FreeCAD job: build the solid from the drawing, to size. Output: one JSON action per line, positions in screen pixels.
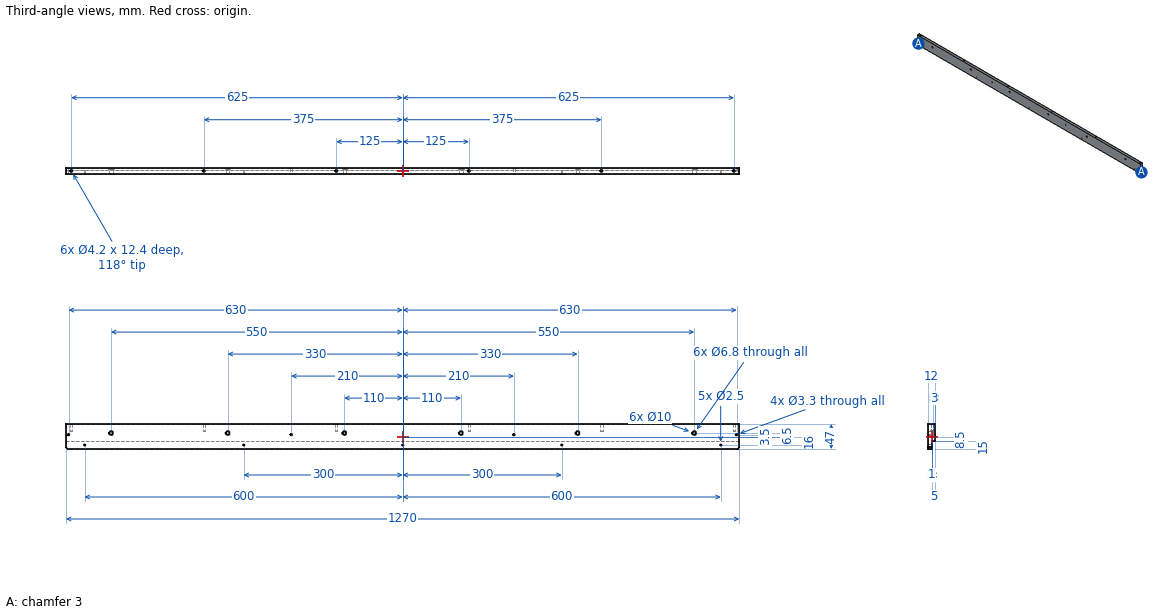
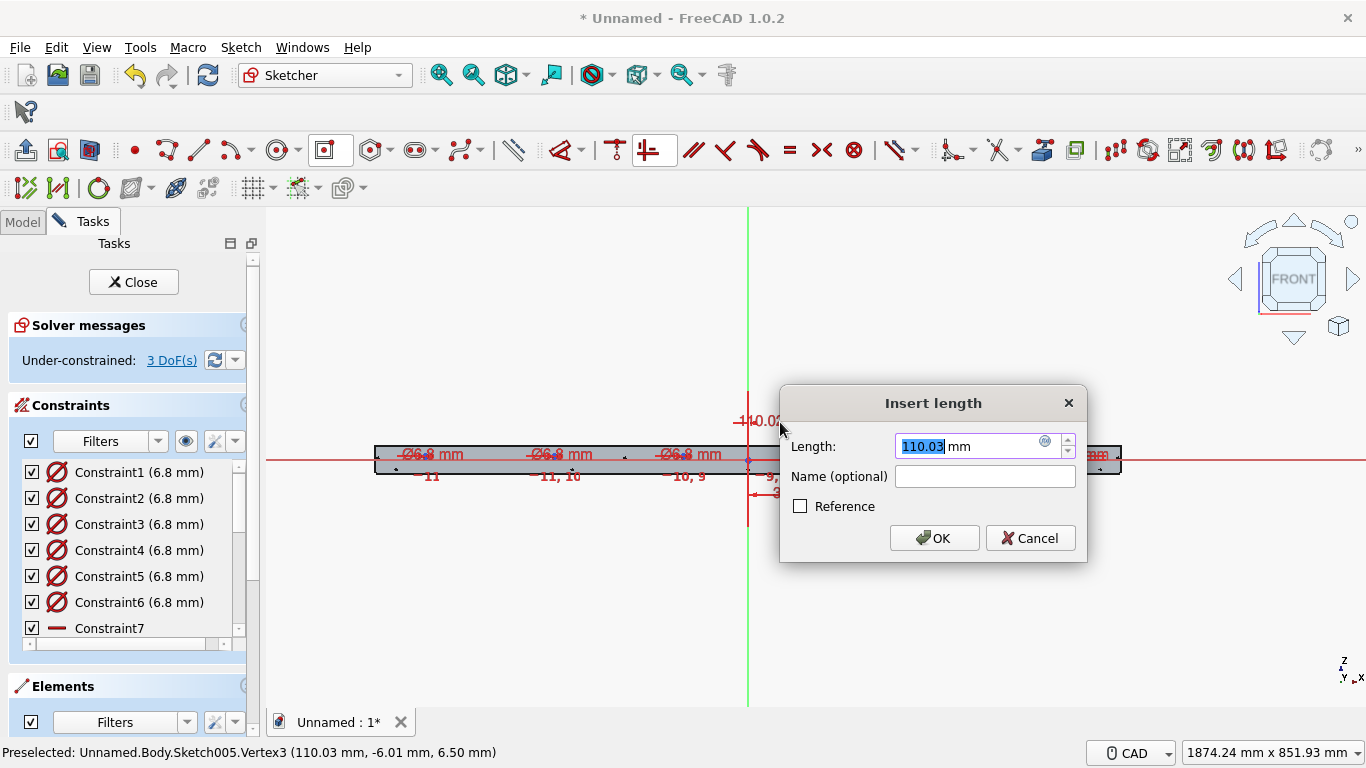
{"action": "type", "text": "110"}
{"action": "key", "text": "Return"}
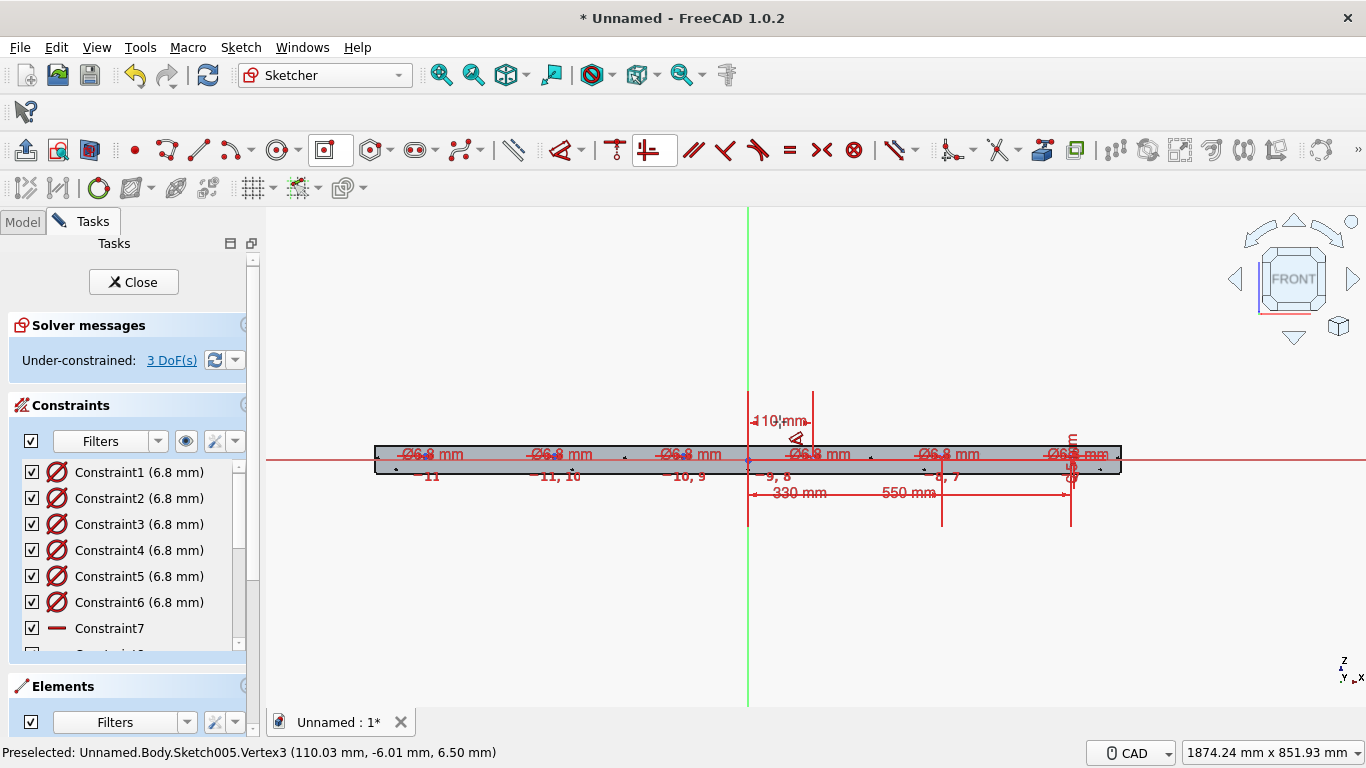
{"action": "left_click", "coordinate": [684, 456]}
{"action": "left_click", "coordinate": [716, 494]}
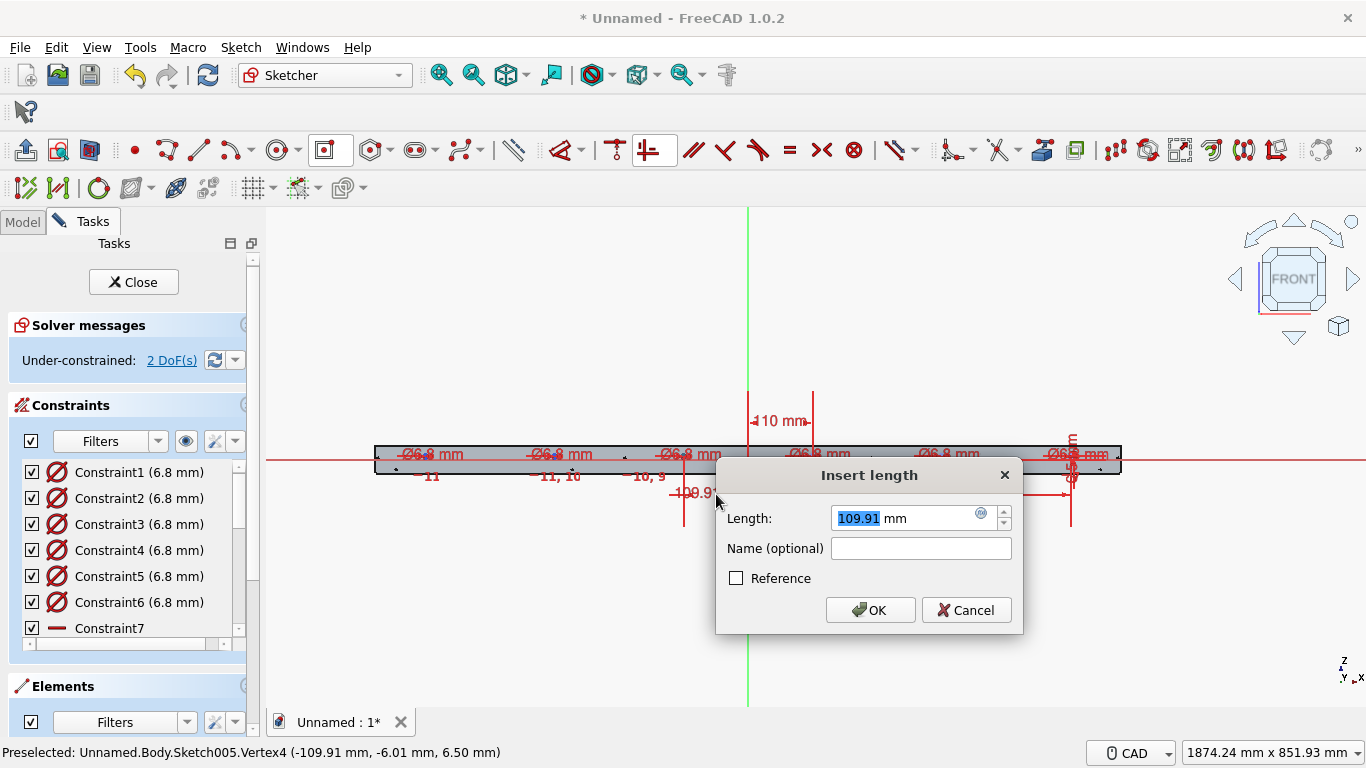
{"action": "type", "text": "110"}
{"action": "key", "text": "Return"}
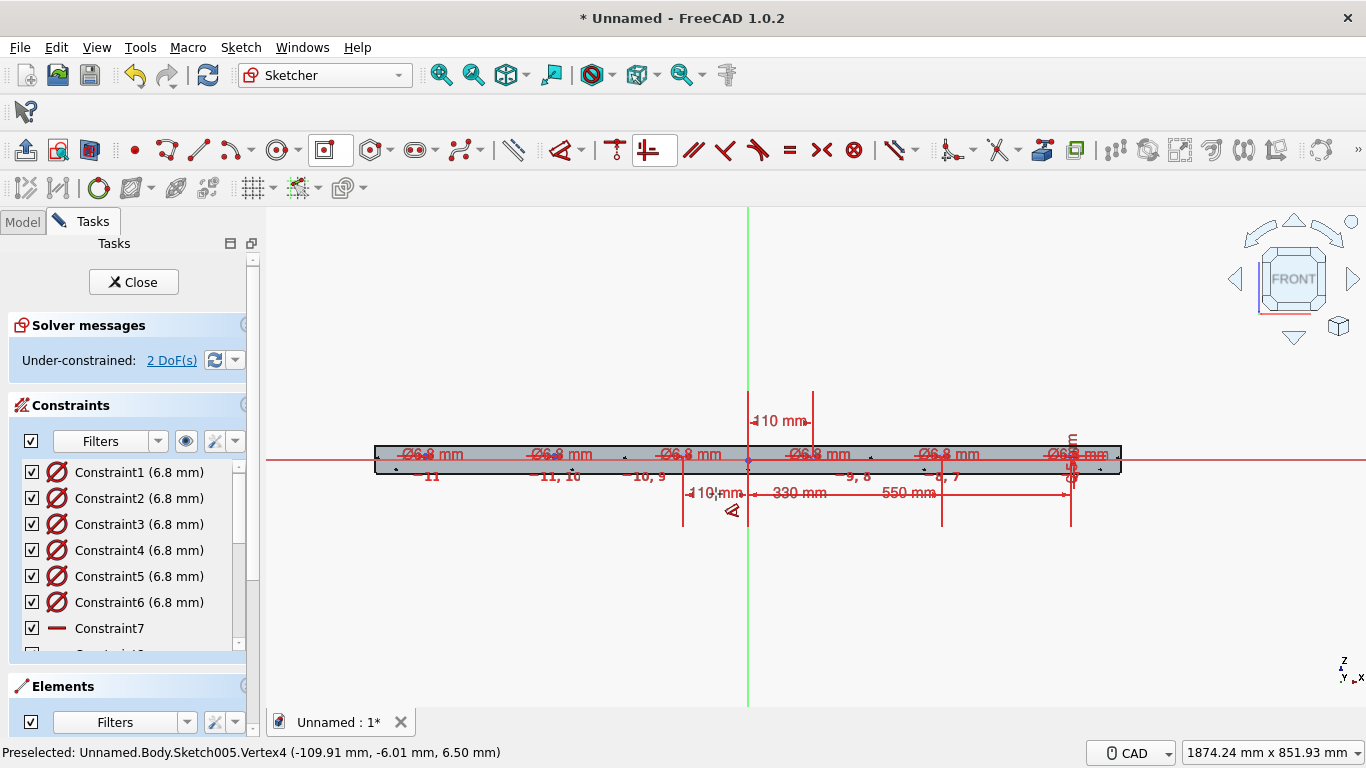
{"action": "left_click", "coordinate": [554, 456]}
{"action": "left_click", "coordinate": [607, 494]}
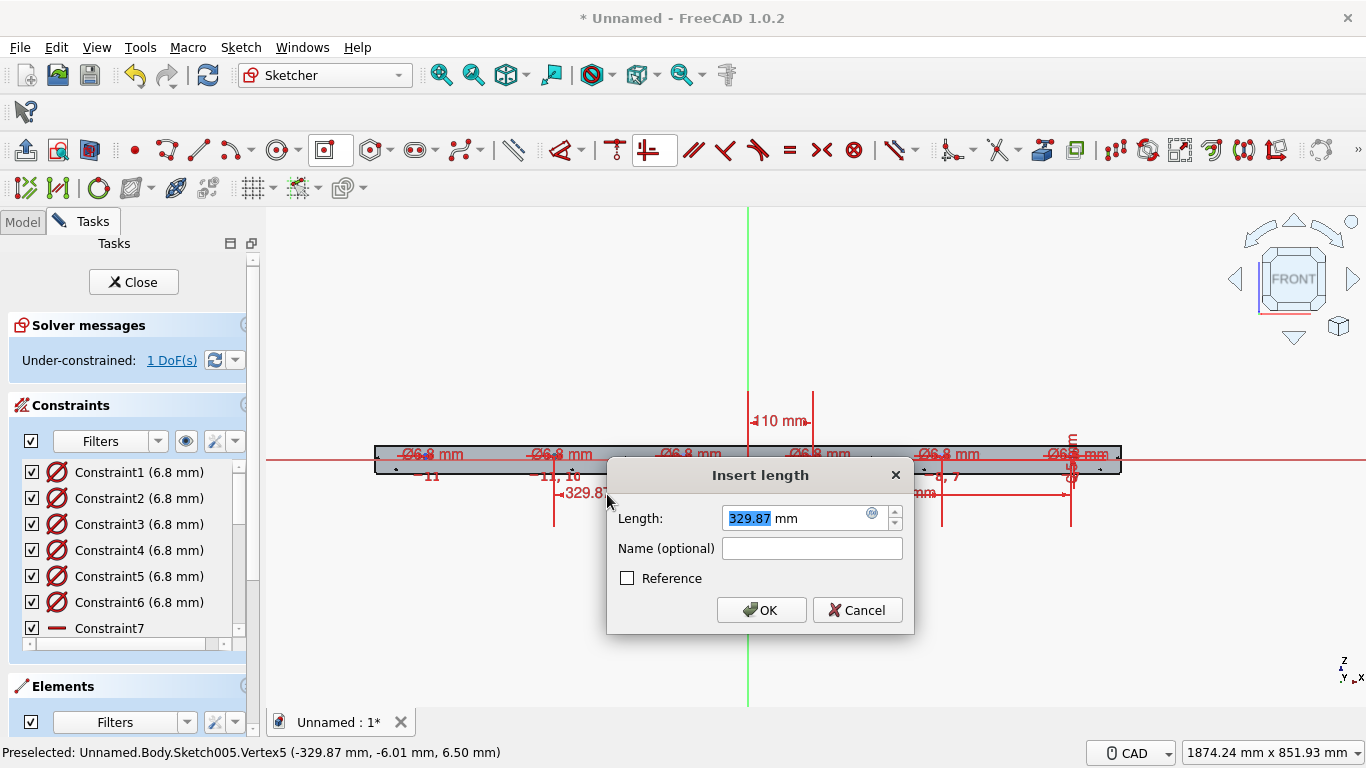
{"action": "type", "text": "330"}
{"action": "key", "text": "Return"}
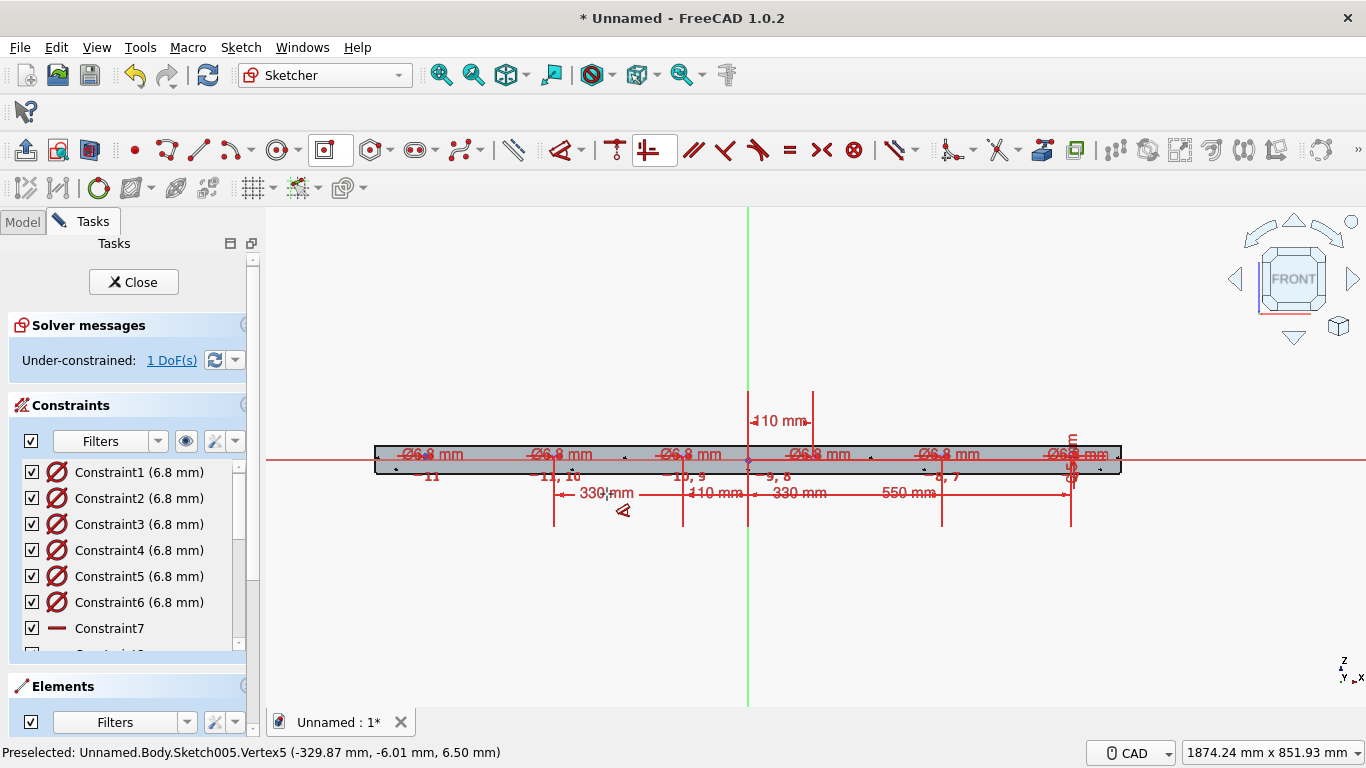
{"action": "left_click", "coordinate": [425, 456]}
{"action": "left_click", "coordinate": [512, 494]}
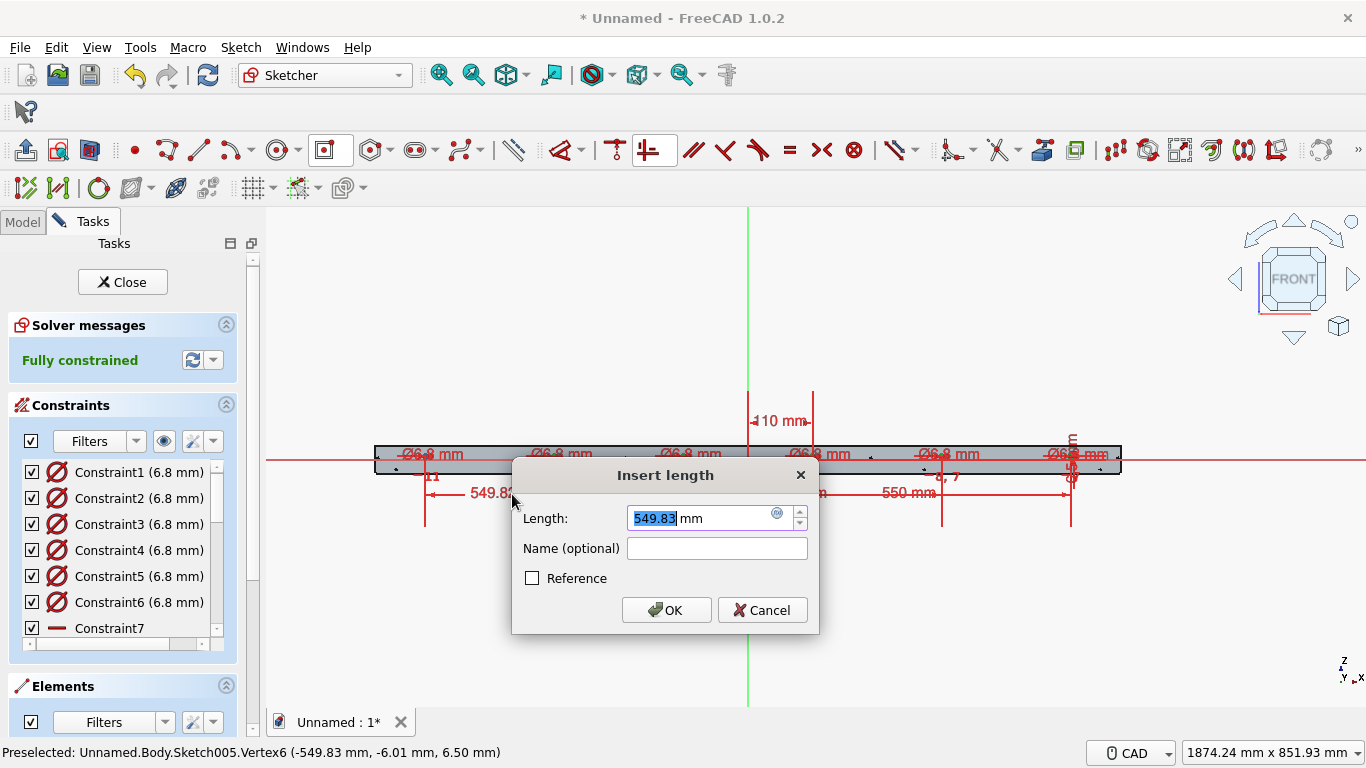
{"action": "type", "text": "550"}
{"action": "key", "text": "Return"}
{"action": "key", "text": "Escape"}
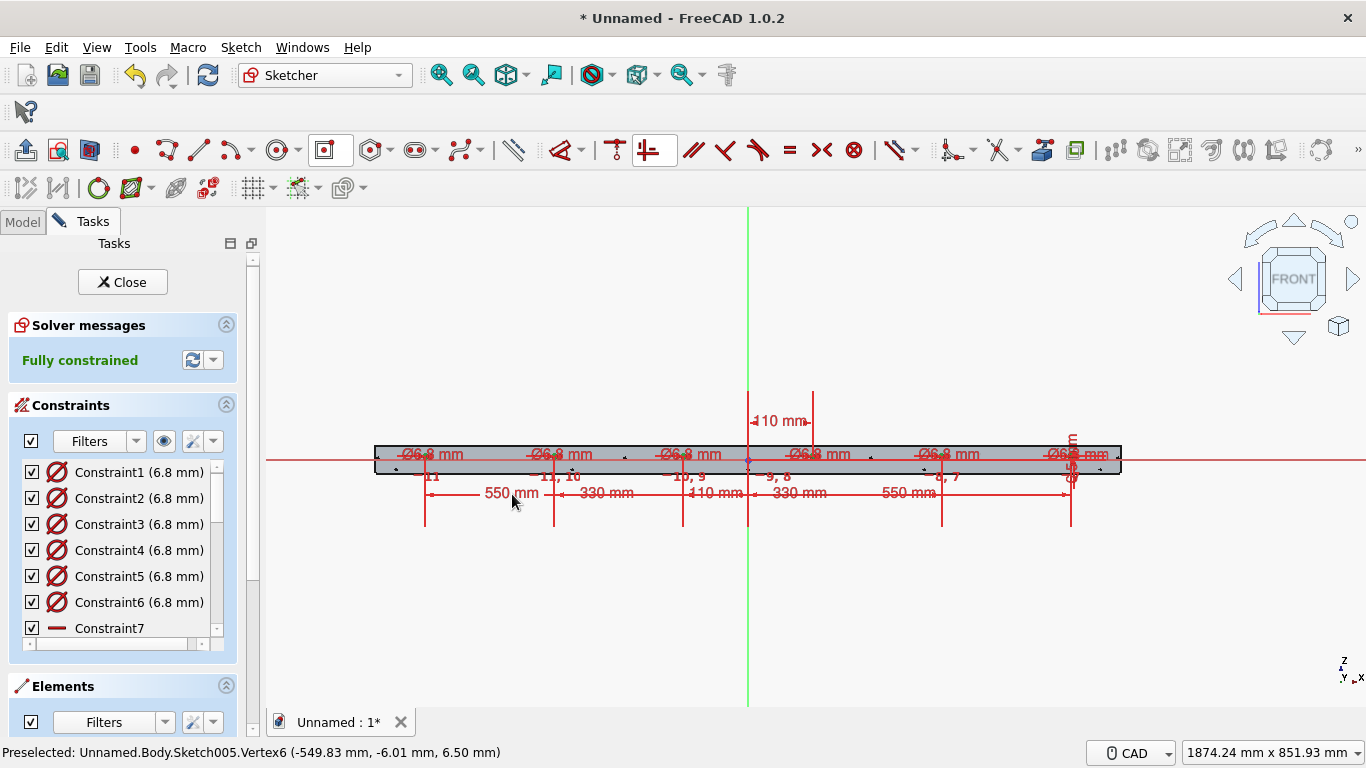
{"action": "left_click", "coordinate": [123, 282]}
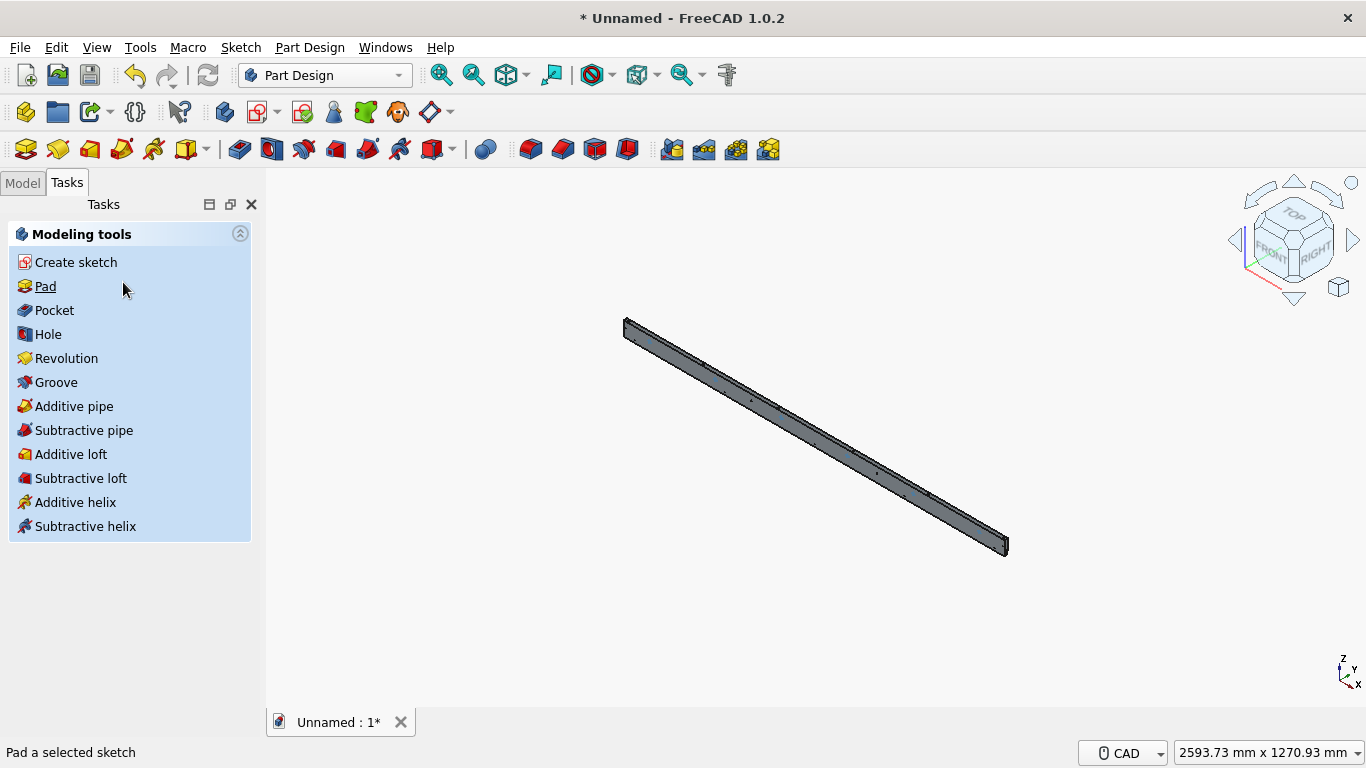
{"action": "left_click", "coordinate": [272, 150]}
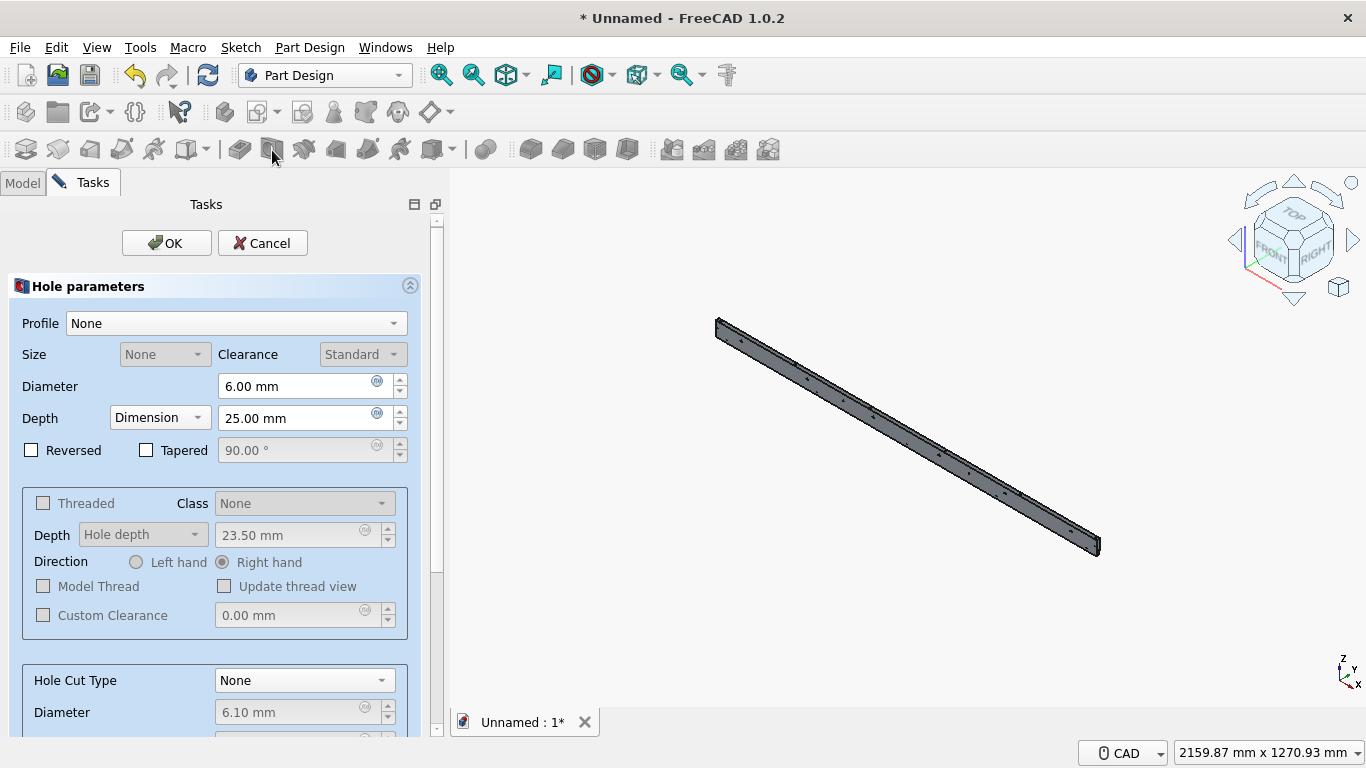
{"action": "triple_click", "coordinate": [305, 386]}